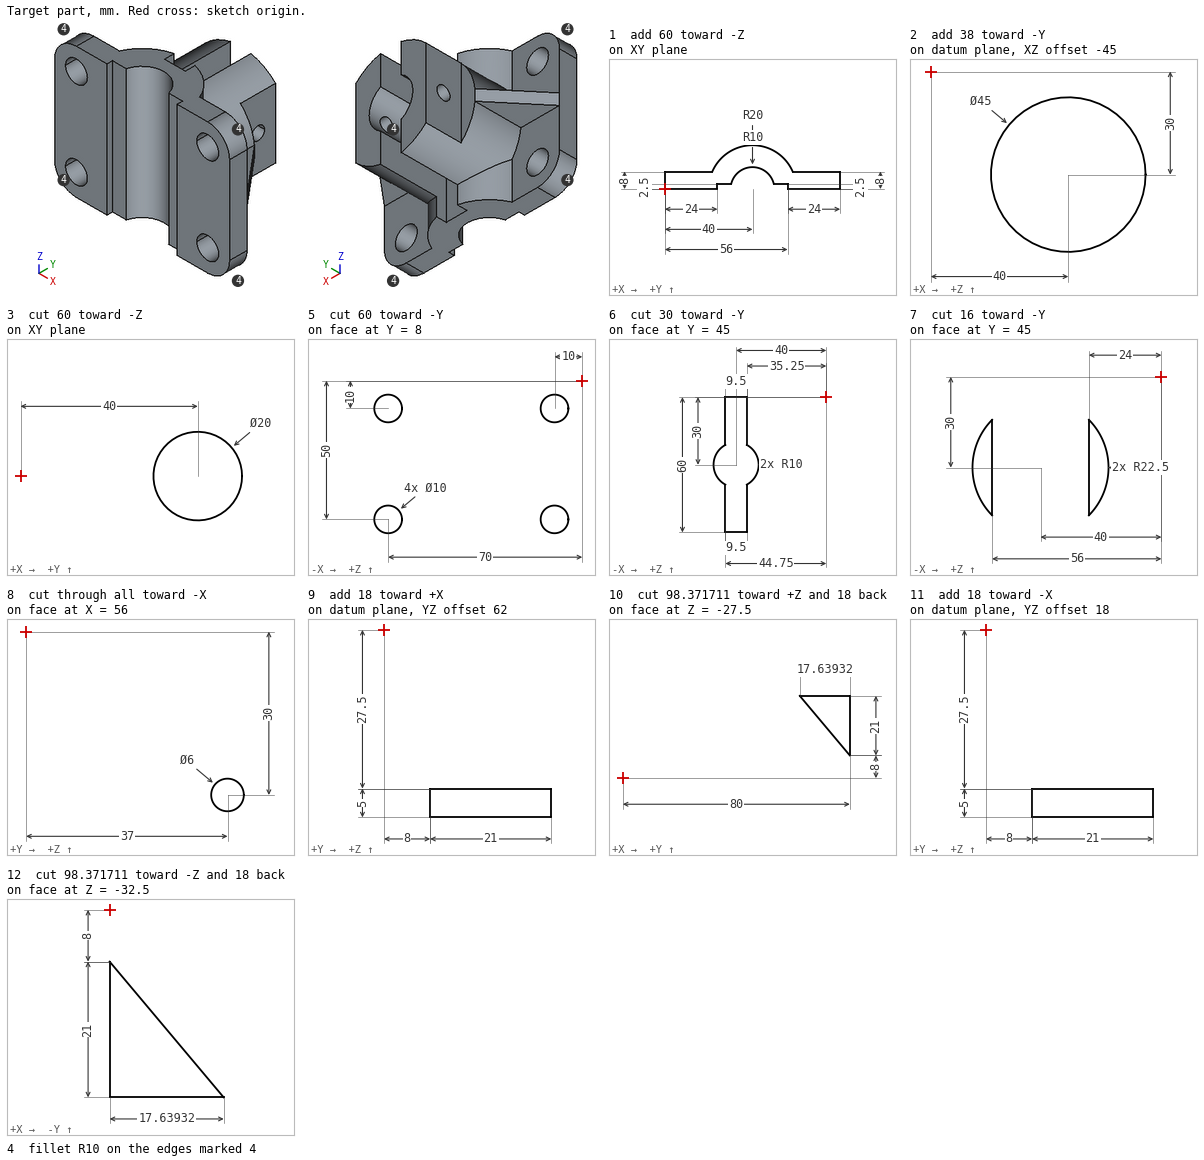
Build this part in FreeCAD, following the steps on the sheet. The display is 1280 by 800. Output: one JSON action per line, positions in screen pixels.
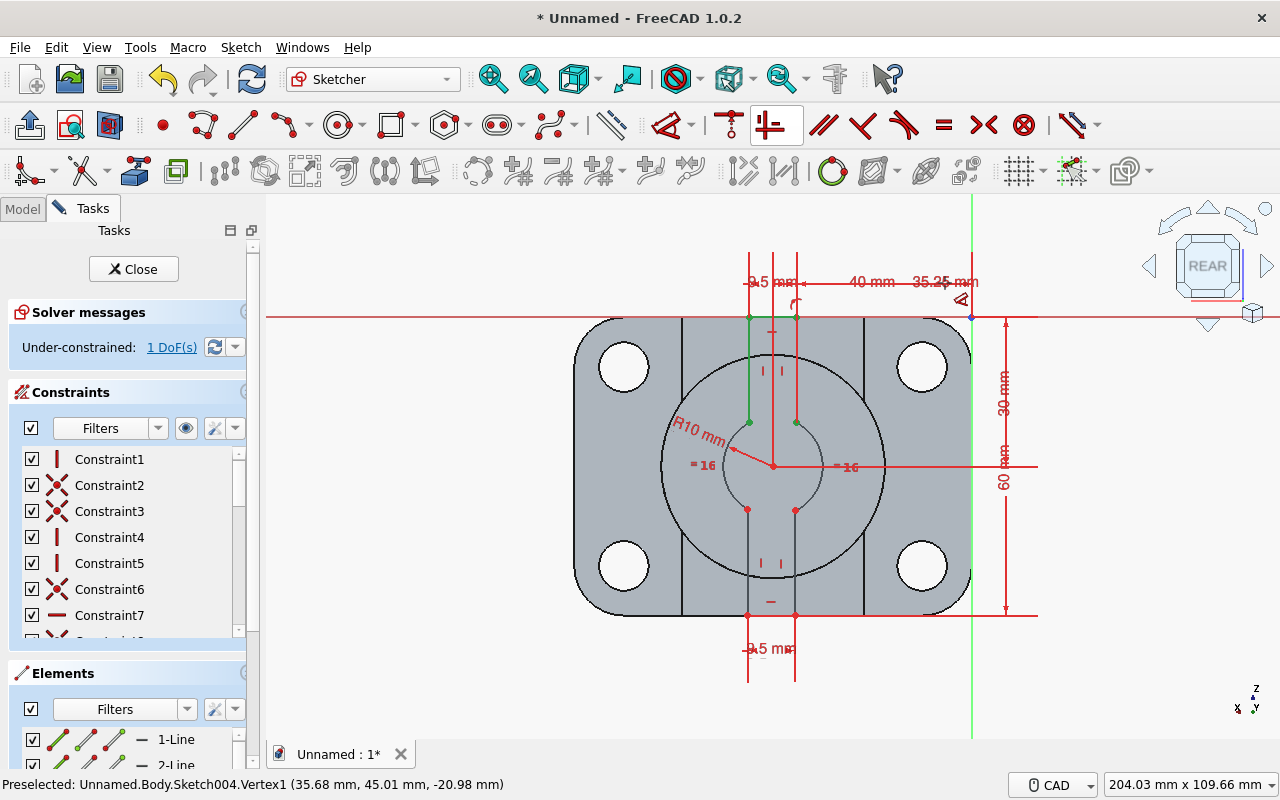
{"action": "left_click", "coordinate": [748, 509]}
{"action": "left_click", "coordinate": [860, 543]}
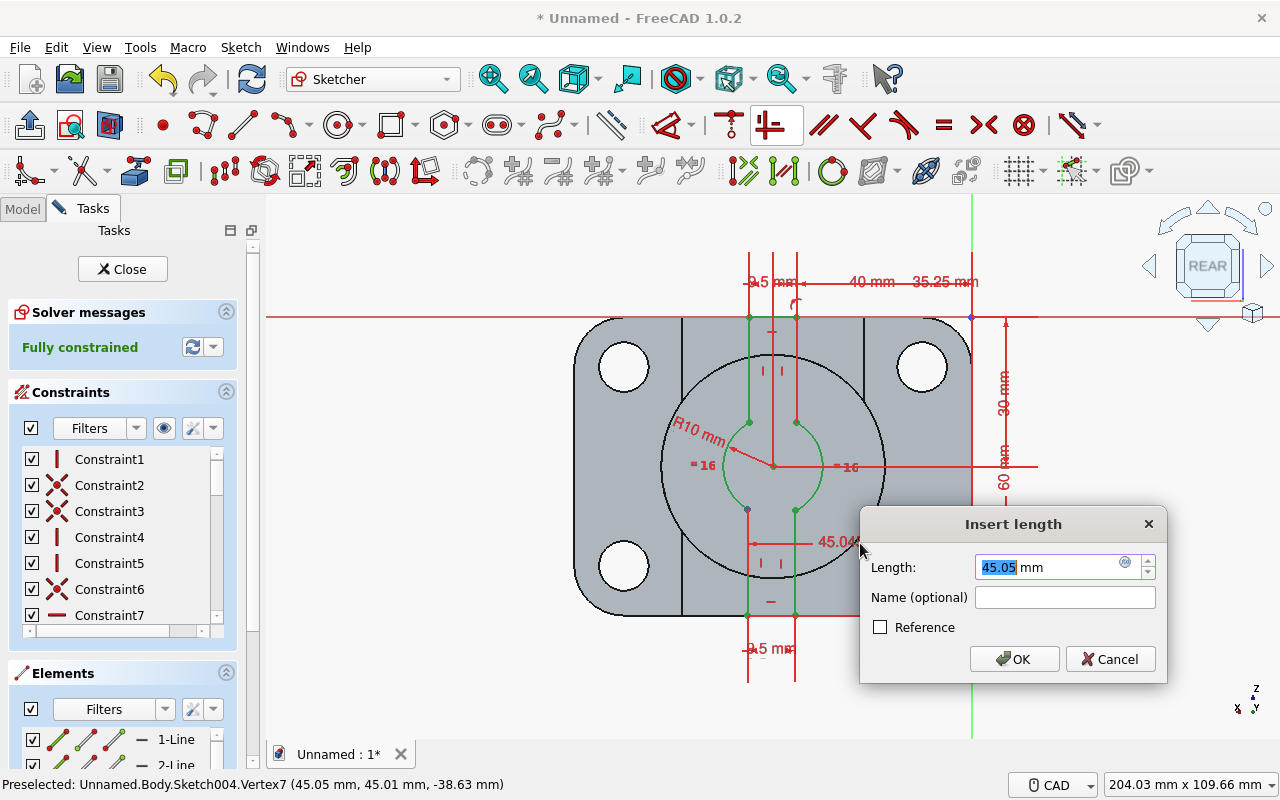
{"action": "type", "text": "44.75"}
{"action": "key", "text": "Return"}
{"action": "key", "text": "Escape"}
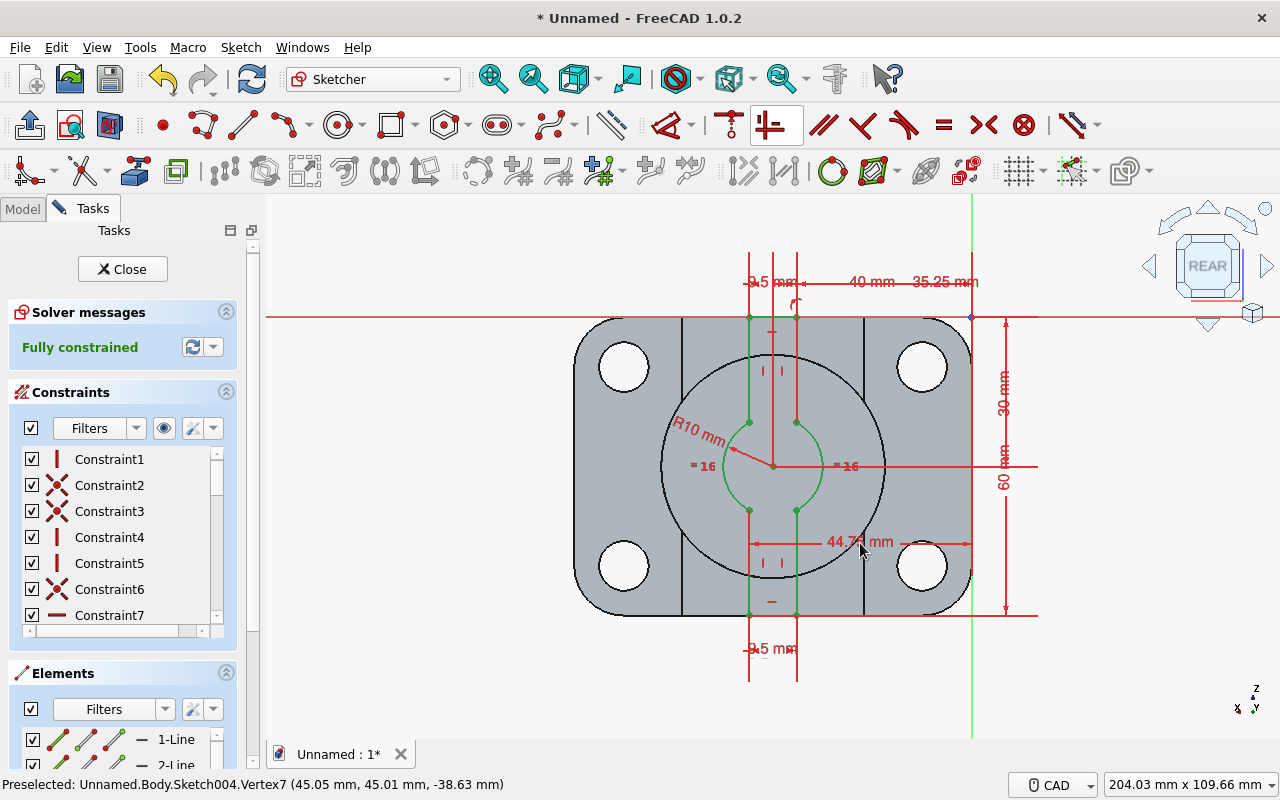
{"action": "left_click", "coordinate": [123, 269]}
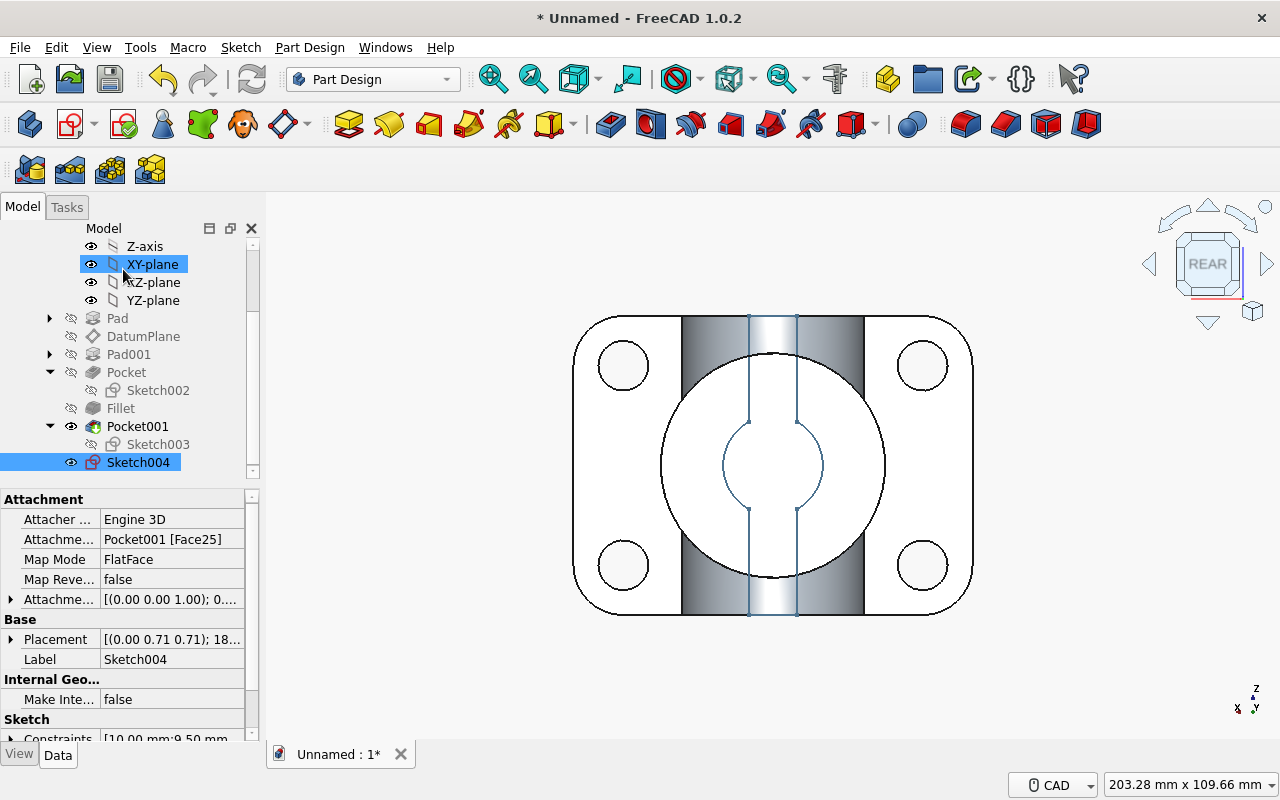
{"action": "left_click", "coordinate": [612, 124]}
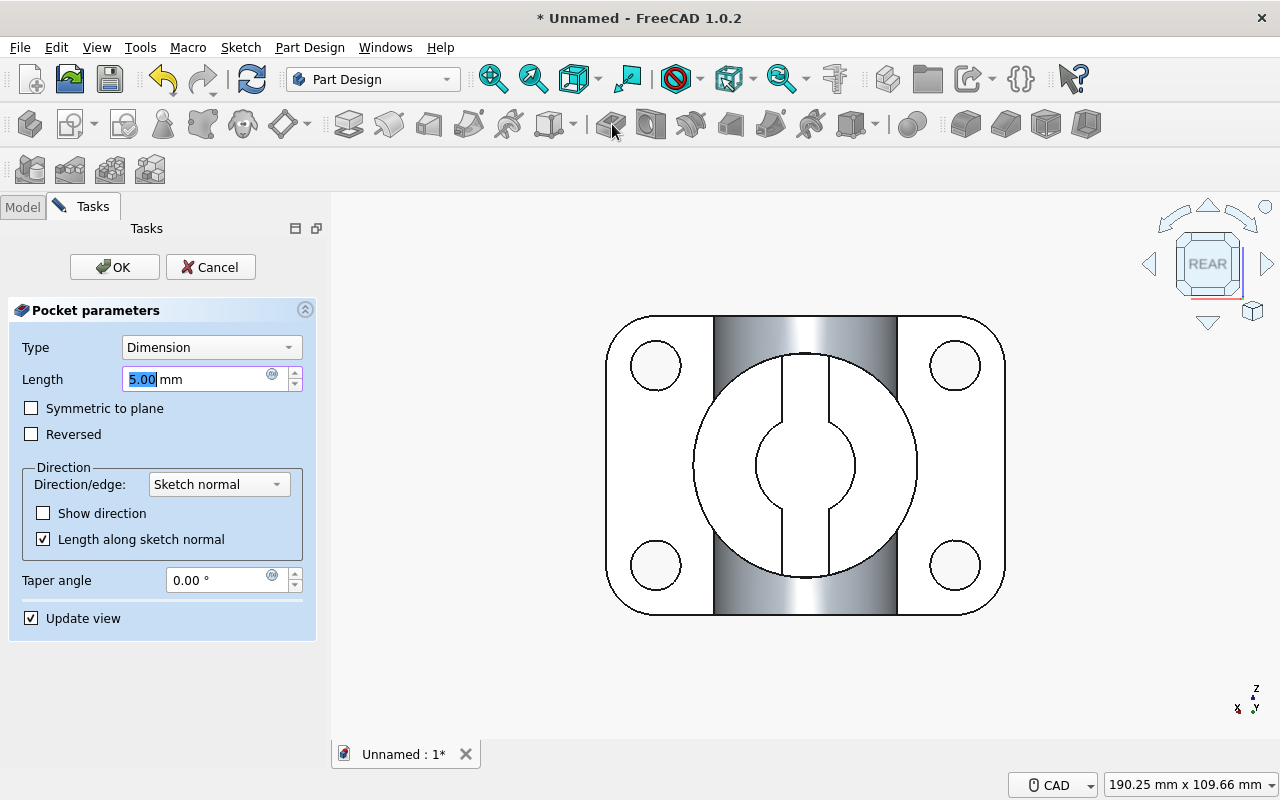
{"action": "type", "text": "30"}
{"action": "key", "text": "Tab"}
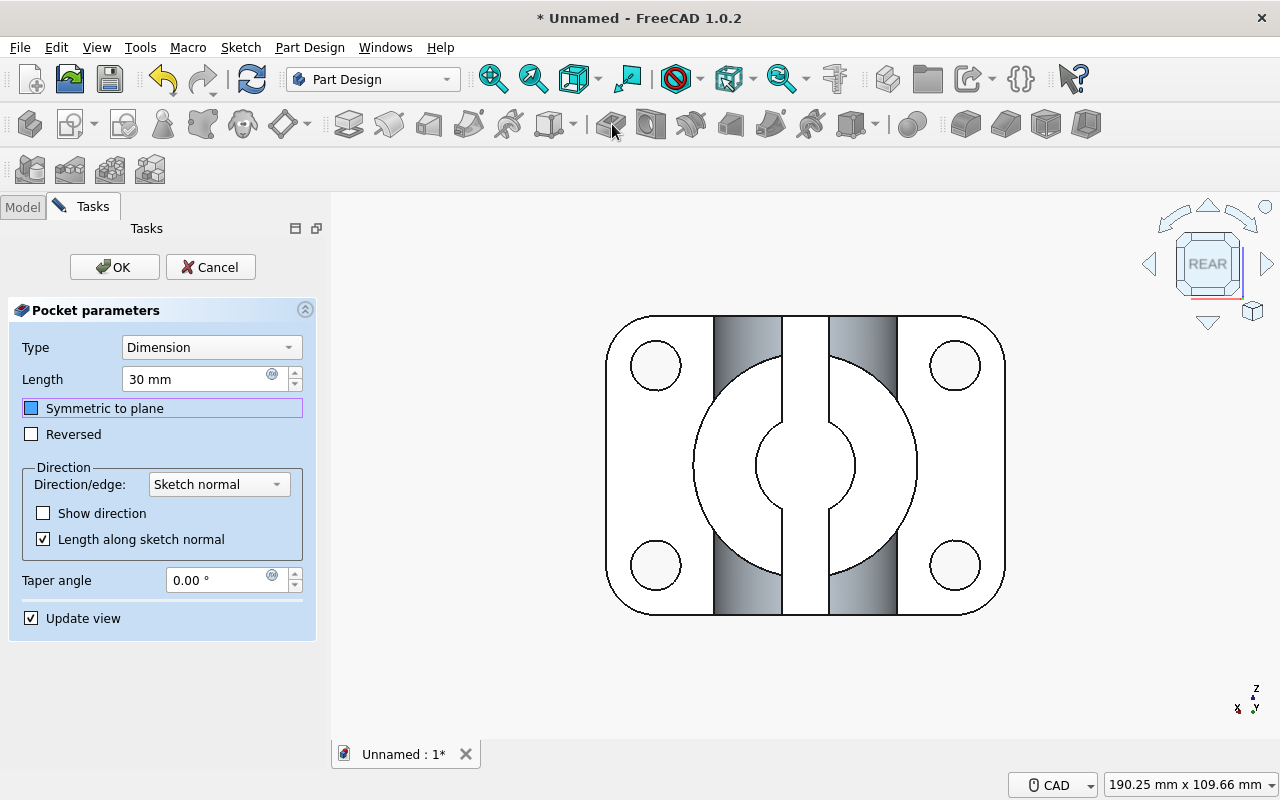
{"action": "left_click", "coordinate": [115, 267]}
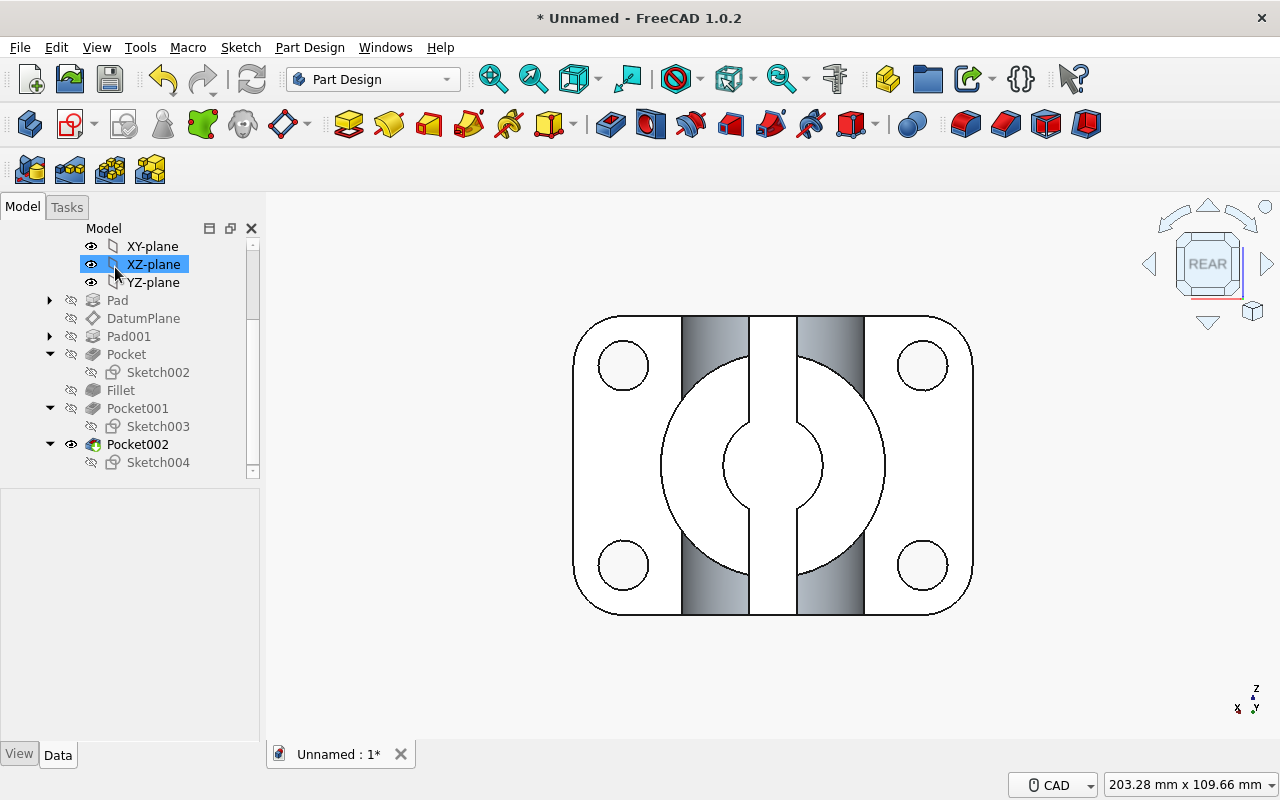
{"action": "left_click", "coordinate": [692, 464]}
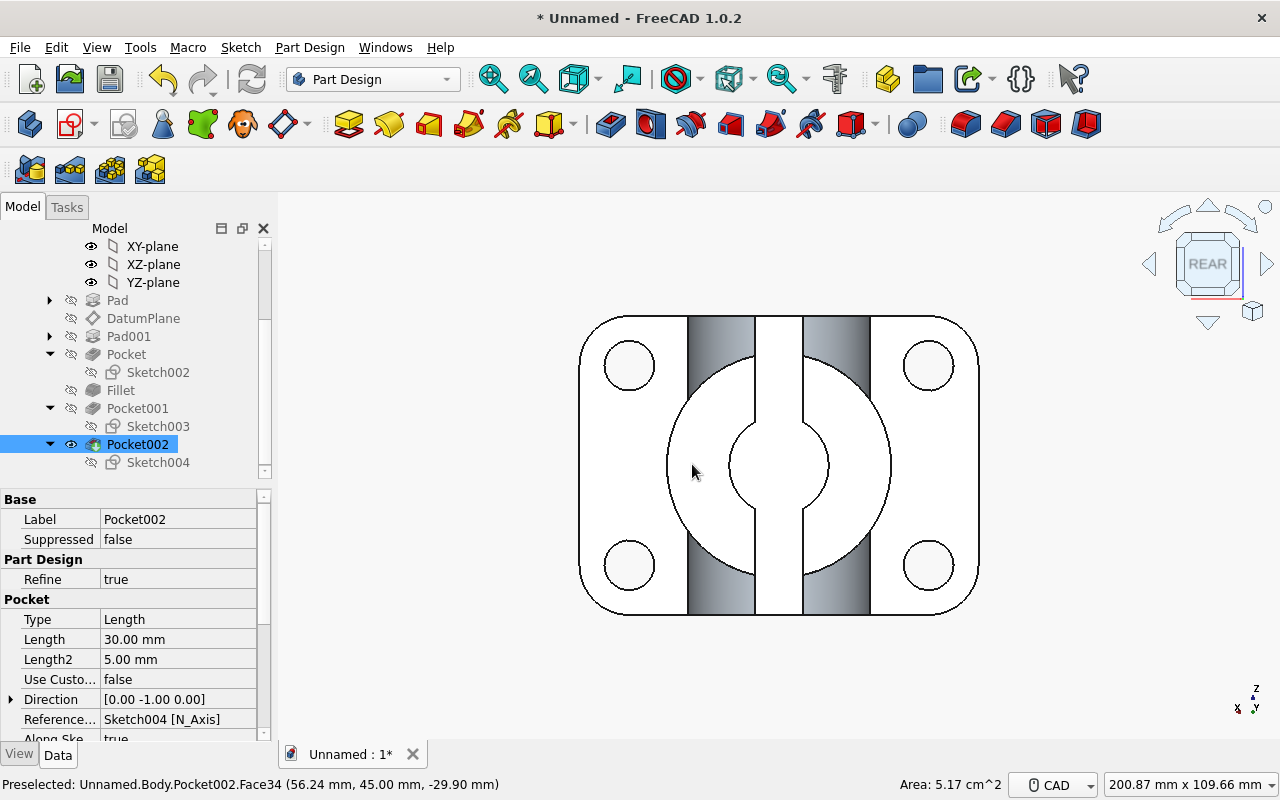
{"action": "left_click", "coordinate": [70, 124]}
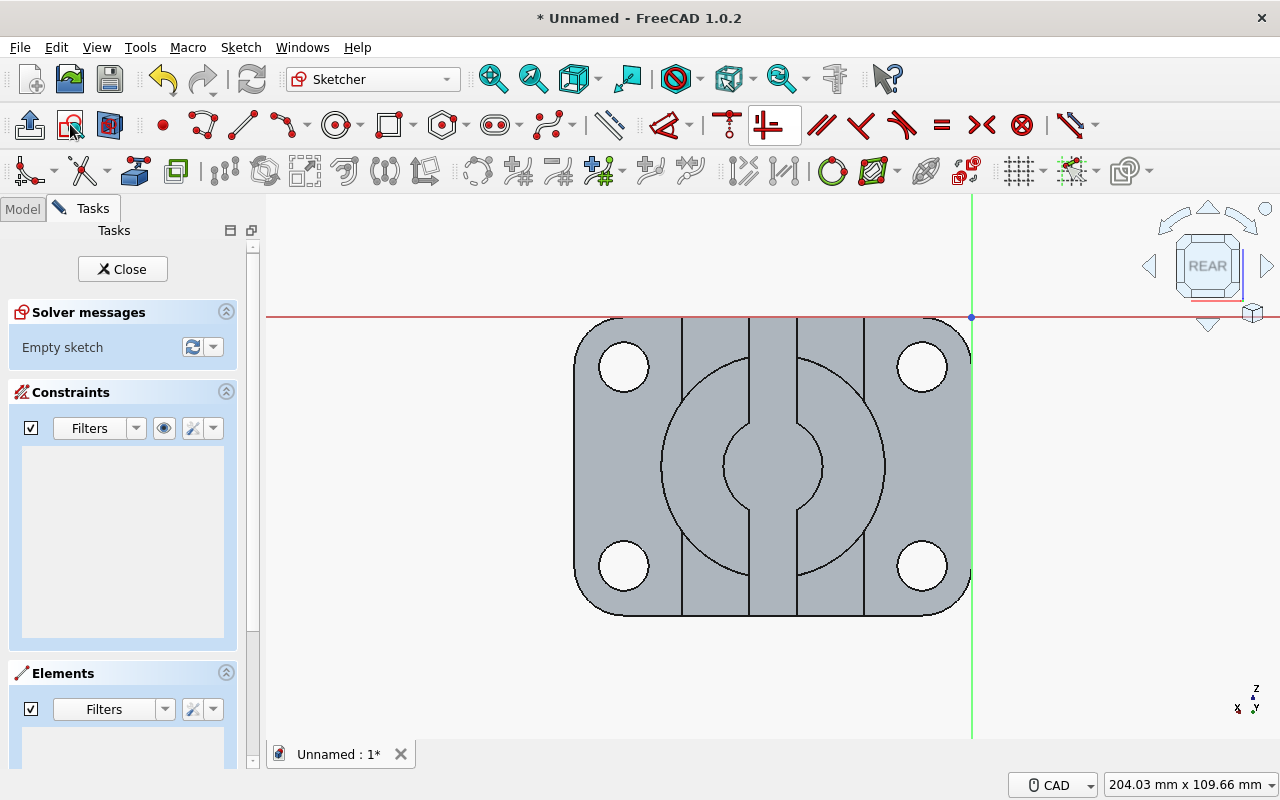
{"action": "scroll", "coordinate": [1044, 360], "scroll_direction": "up", "scroll_amount": 2}